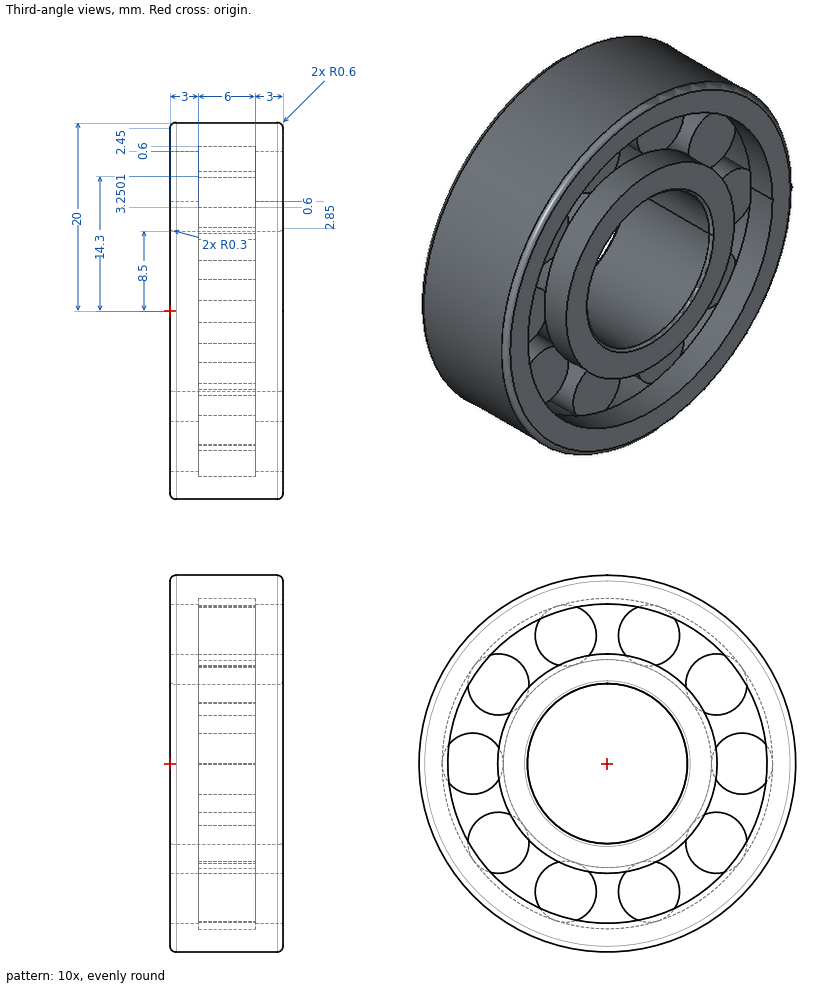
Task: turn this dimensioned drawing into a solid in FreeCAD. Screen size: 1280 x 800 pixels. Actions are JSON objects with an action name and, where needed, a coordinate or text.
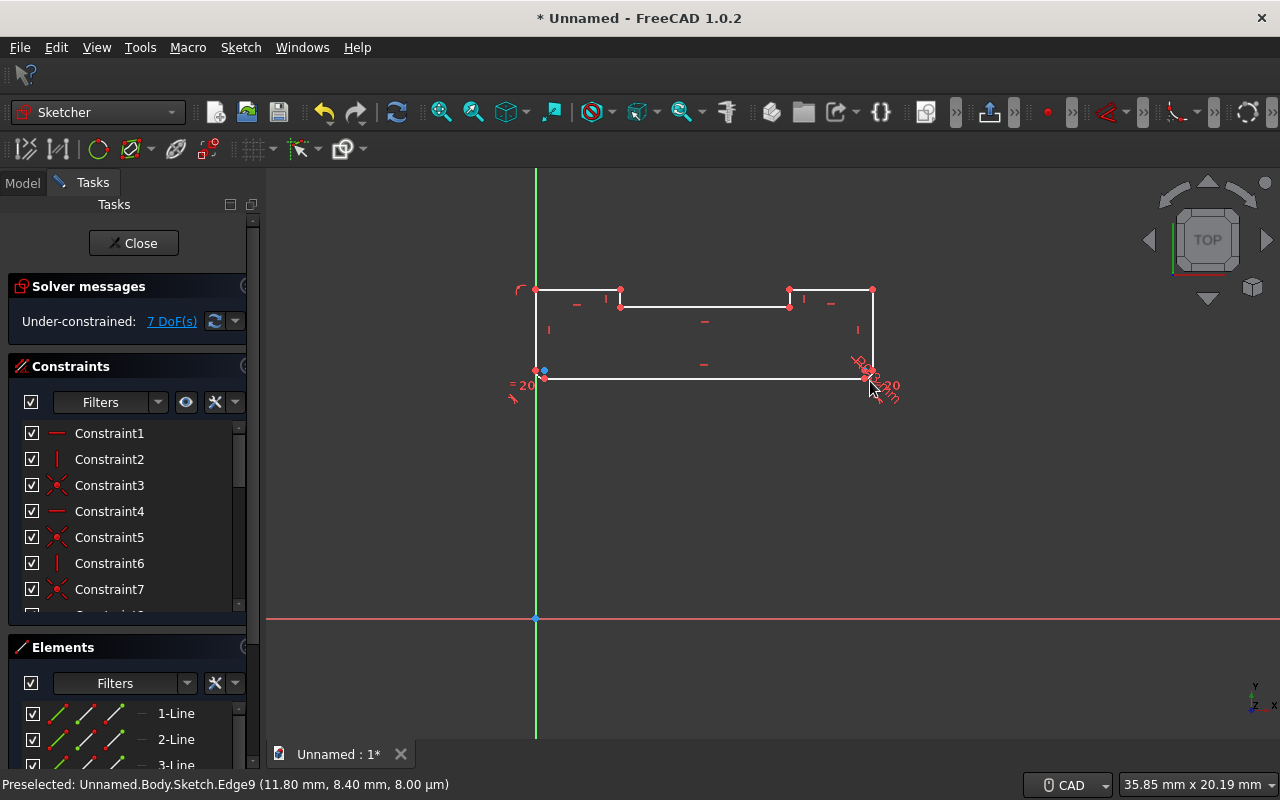
{"action": "left_click", "coordinate": [848, 290]}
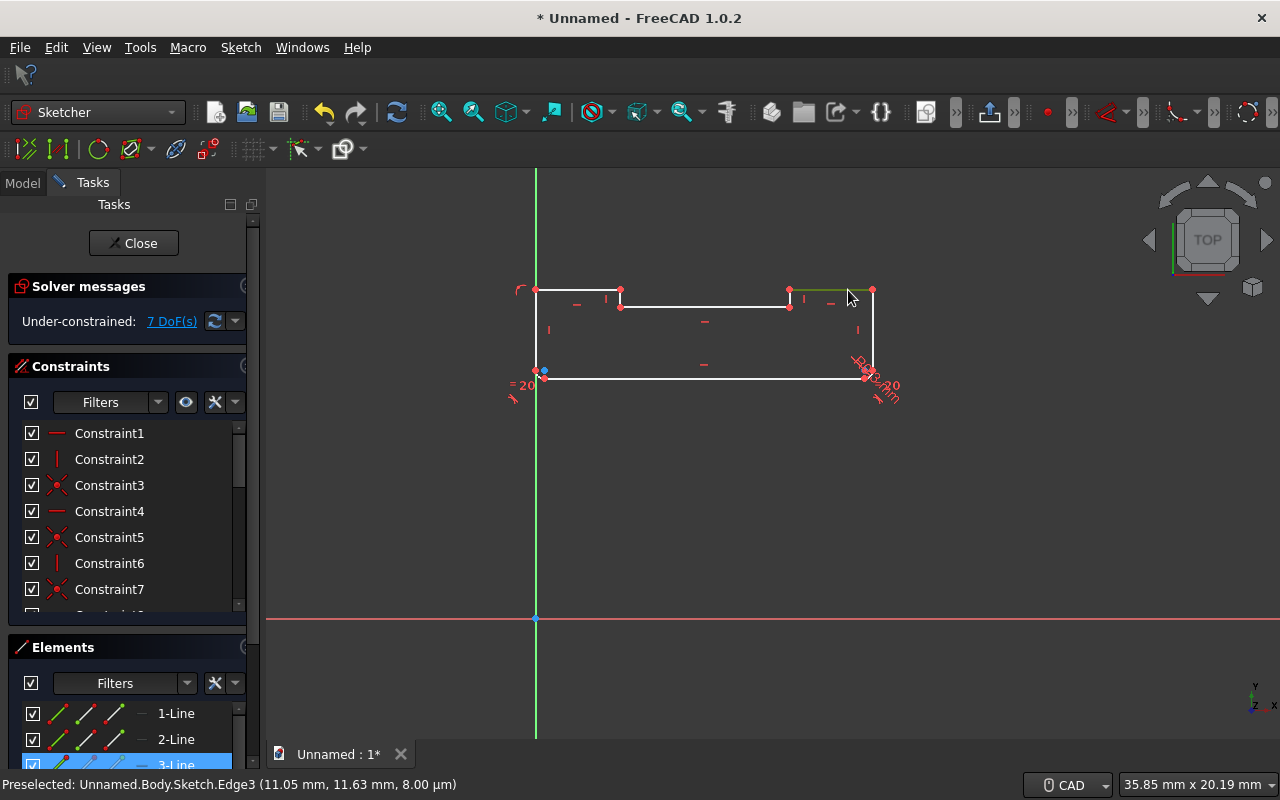
{"action": "key", "text": "l"}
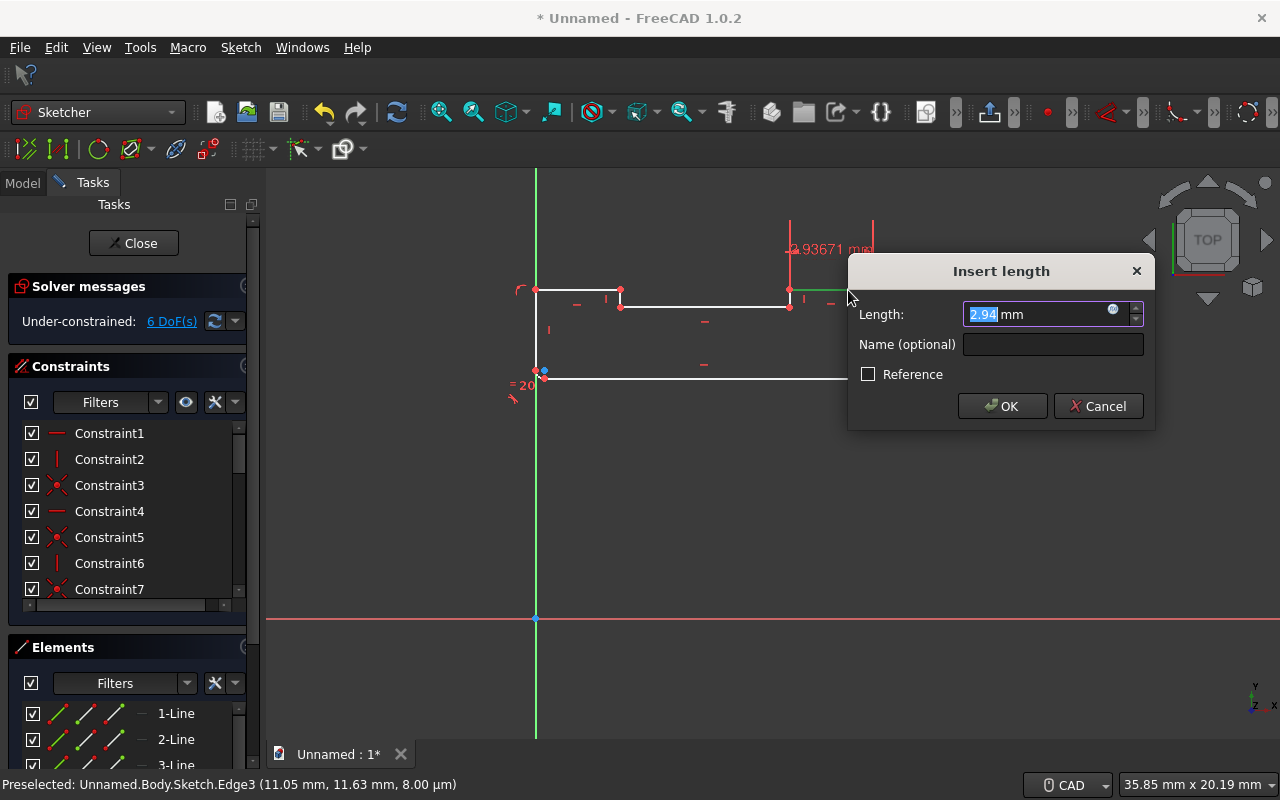
{"action": "type", "text": "3"}
{"action": "key", "text": "Return"}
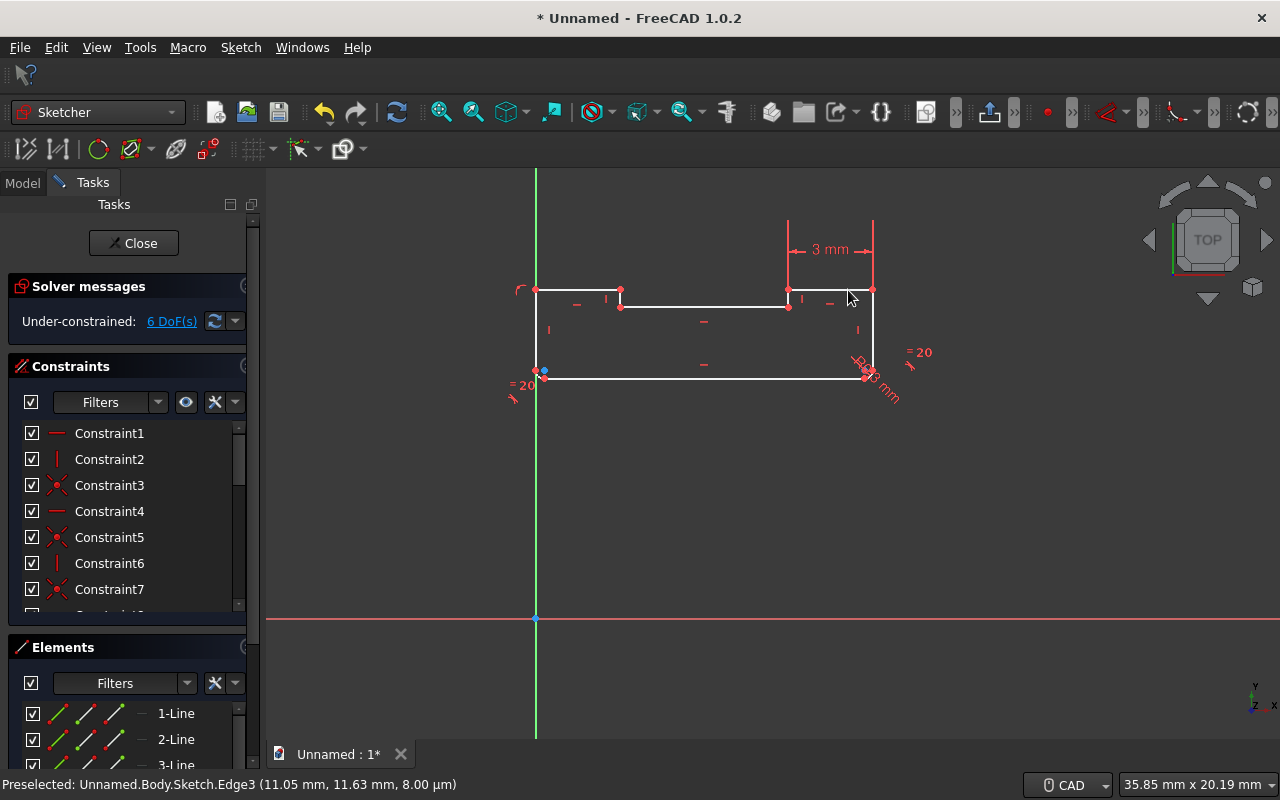
{"action": "left_click", "coordinate": [738, 307]}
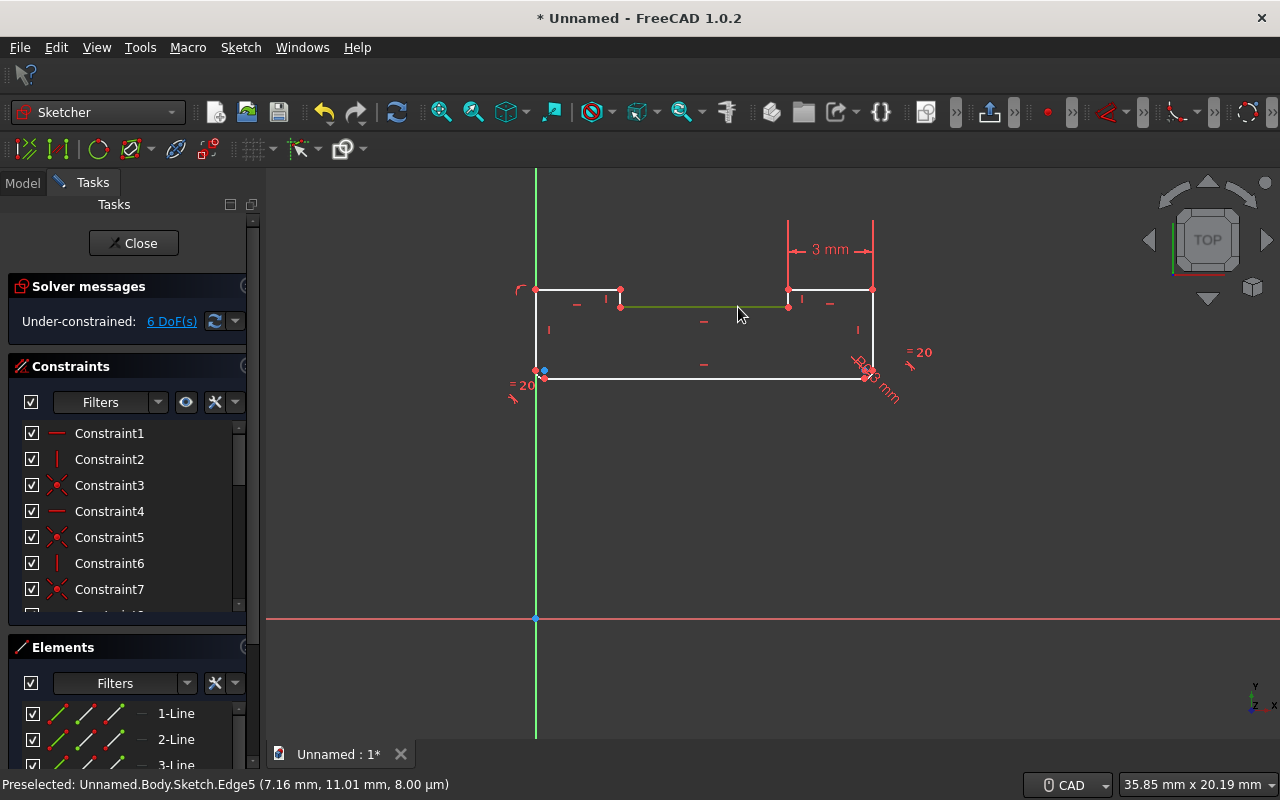
{"action": "left_click", "coordinate": [1128, 112]}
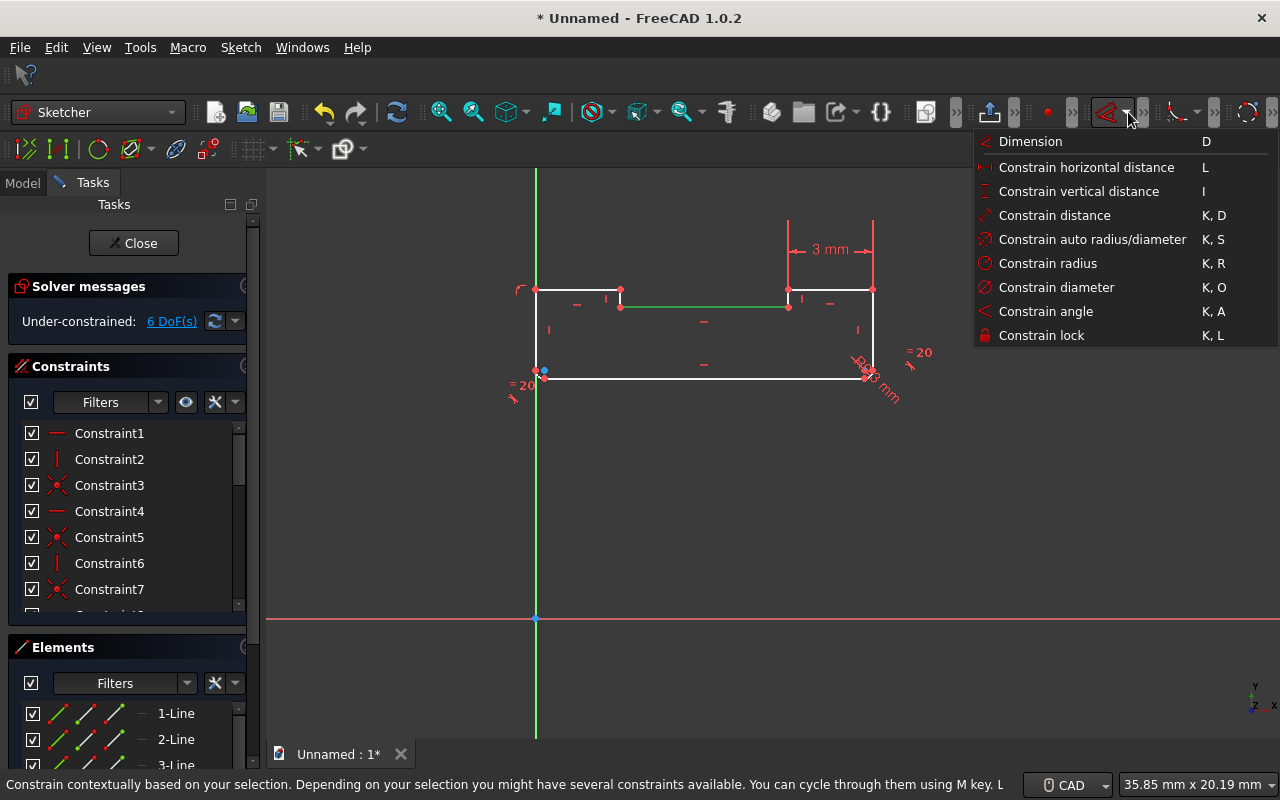
{"action": "left_click", "coordinate": [1126, 167]}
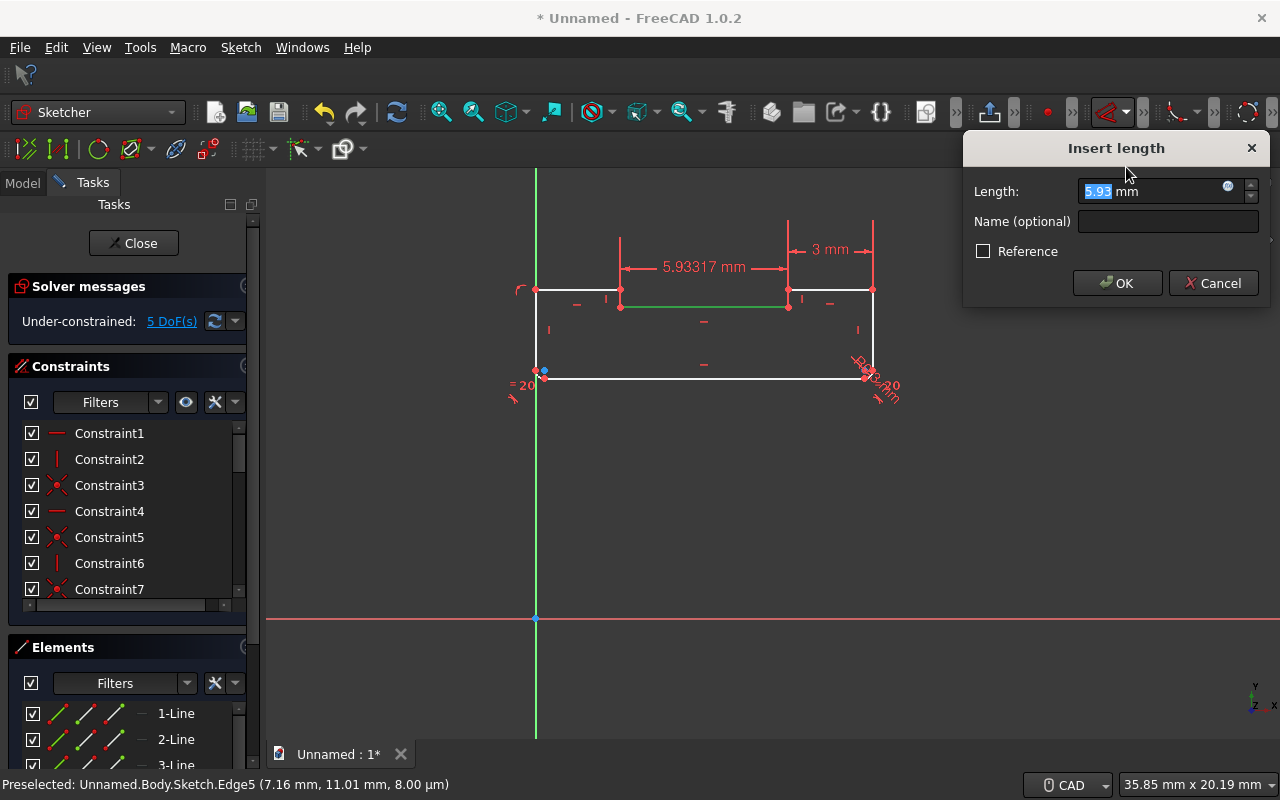
{"action": "type", "text": "6"}
{"action": "key", "text": "Return"}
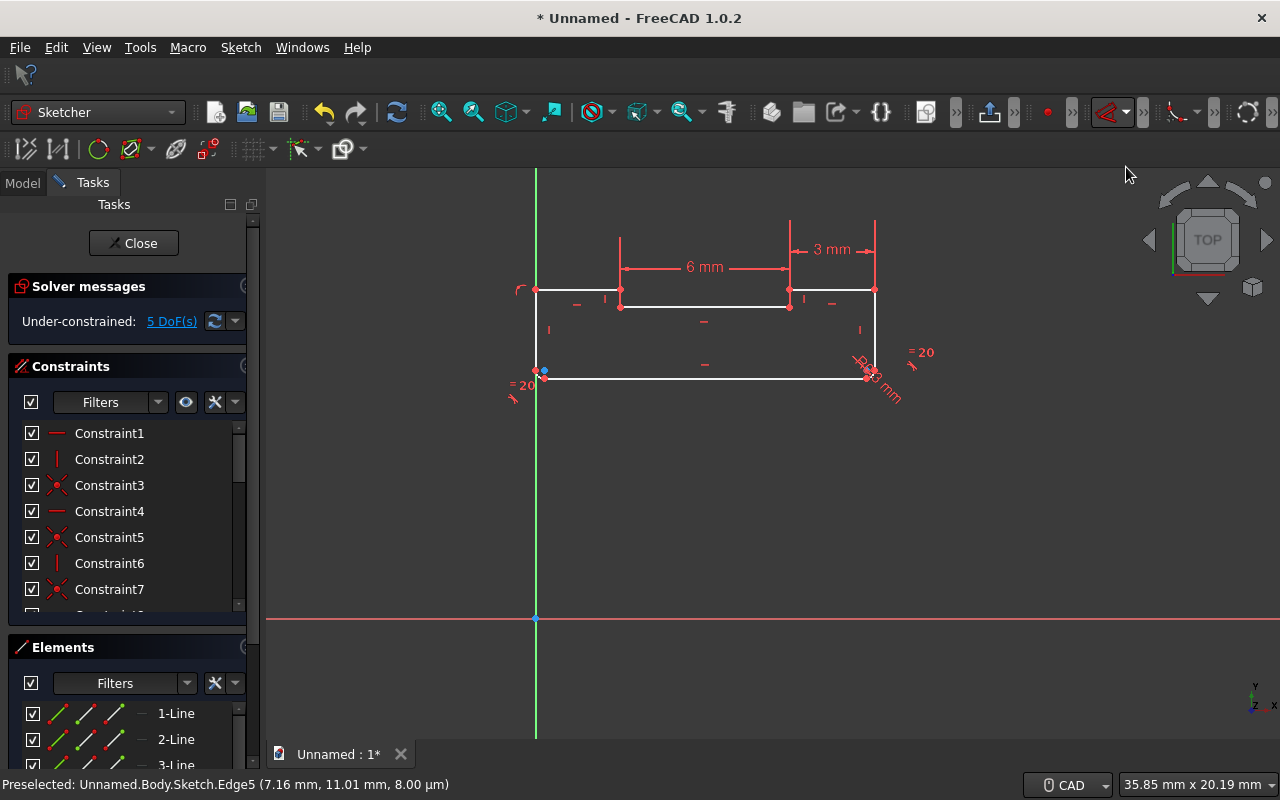
{"action": "left_click", "coordinate": [595, 290]}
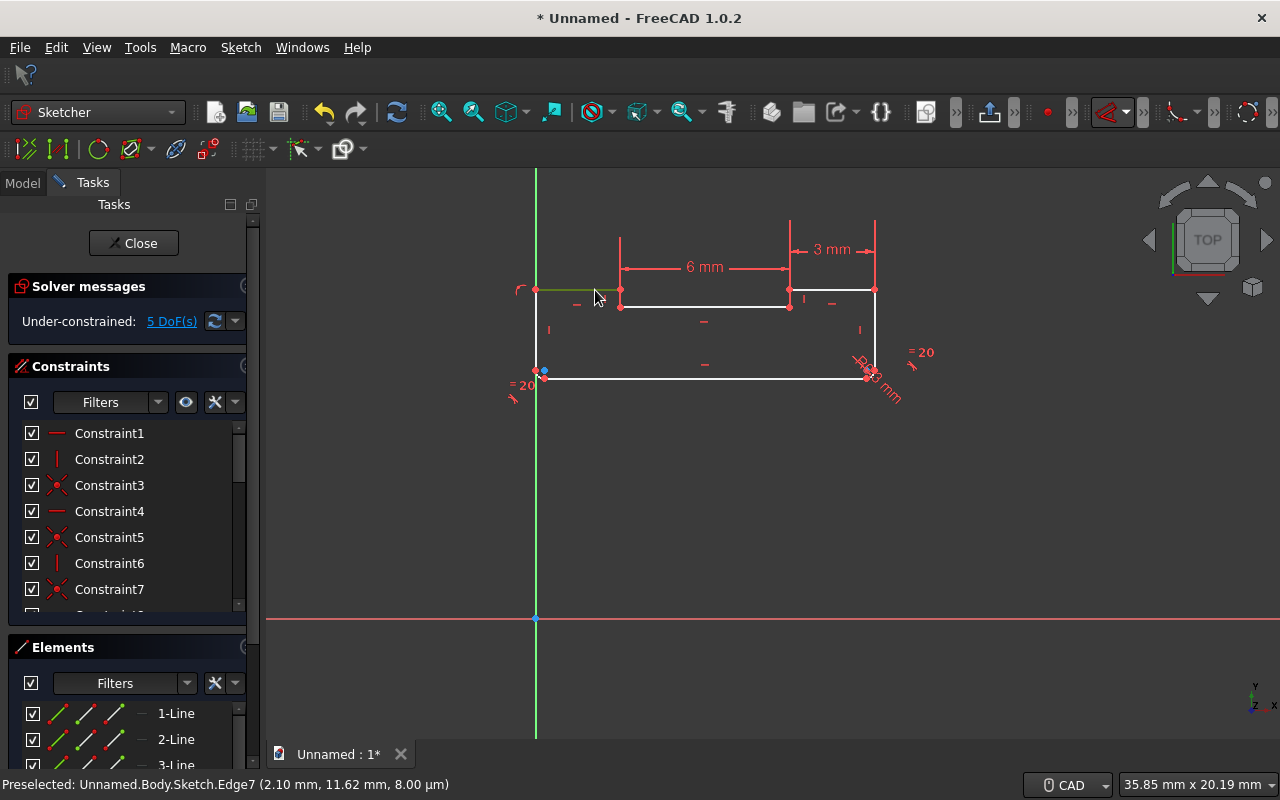
{"action": "left_click", "coordinate": [1128, 112]}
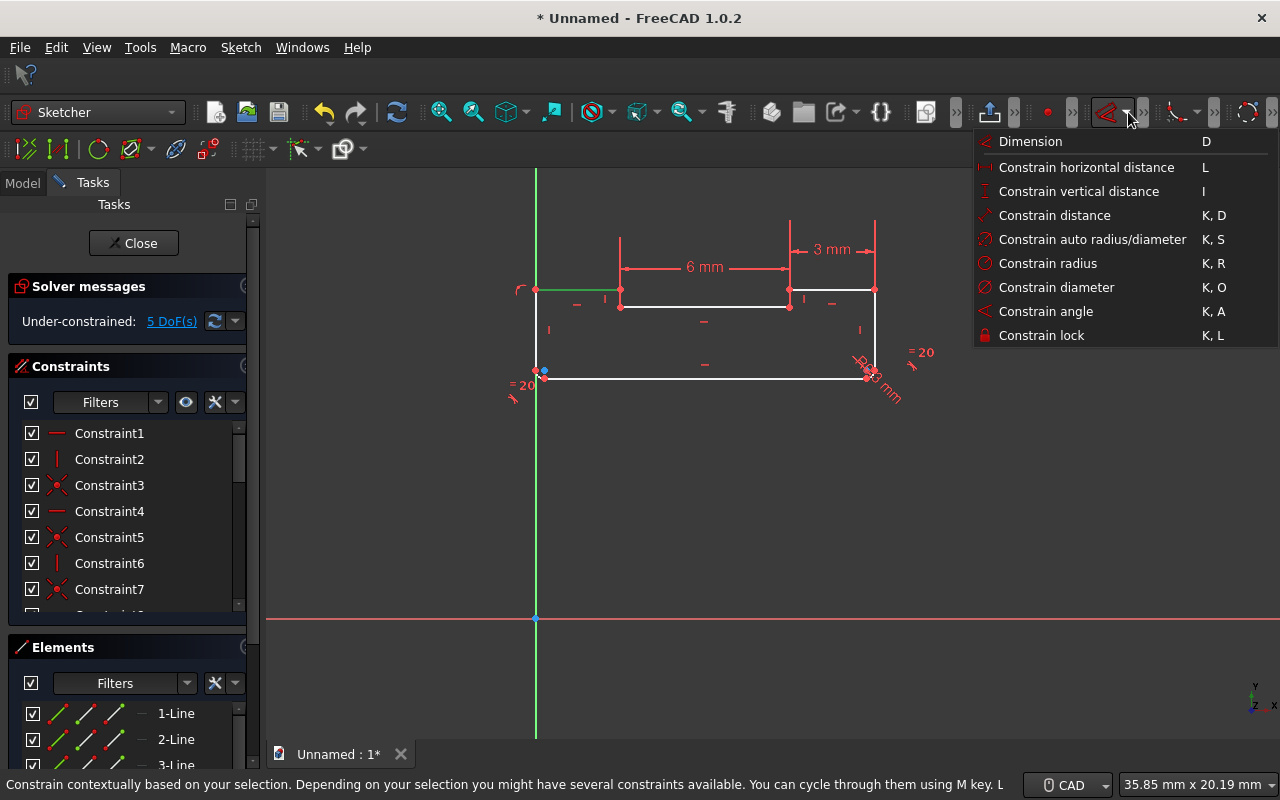
{"action": "left_click", "coordinate": [1126, 167]}